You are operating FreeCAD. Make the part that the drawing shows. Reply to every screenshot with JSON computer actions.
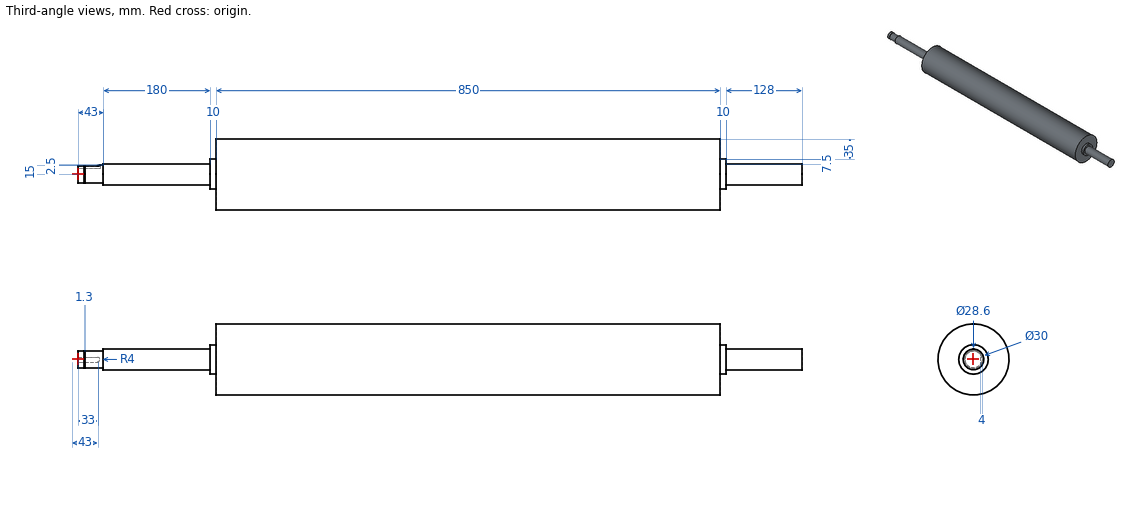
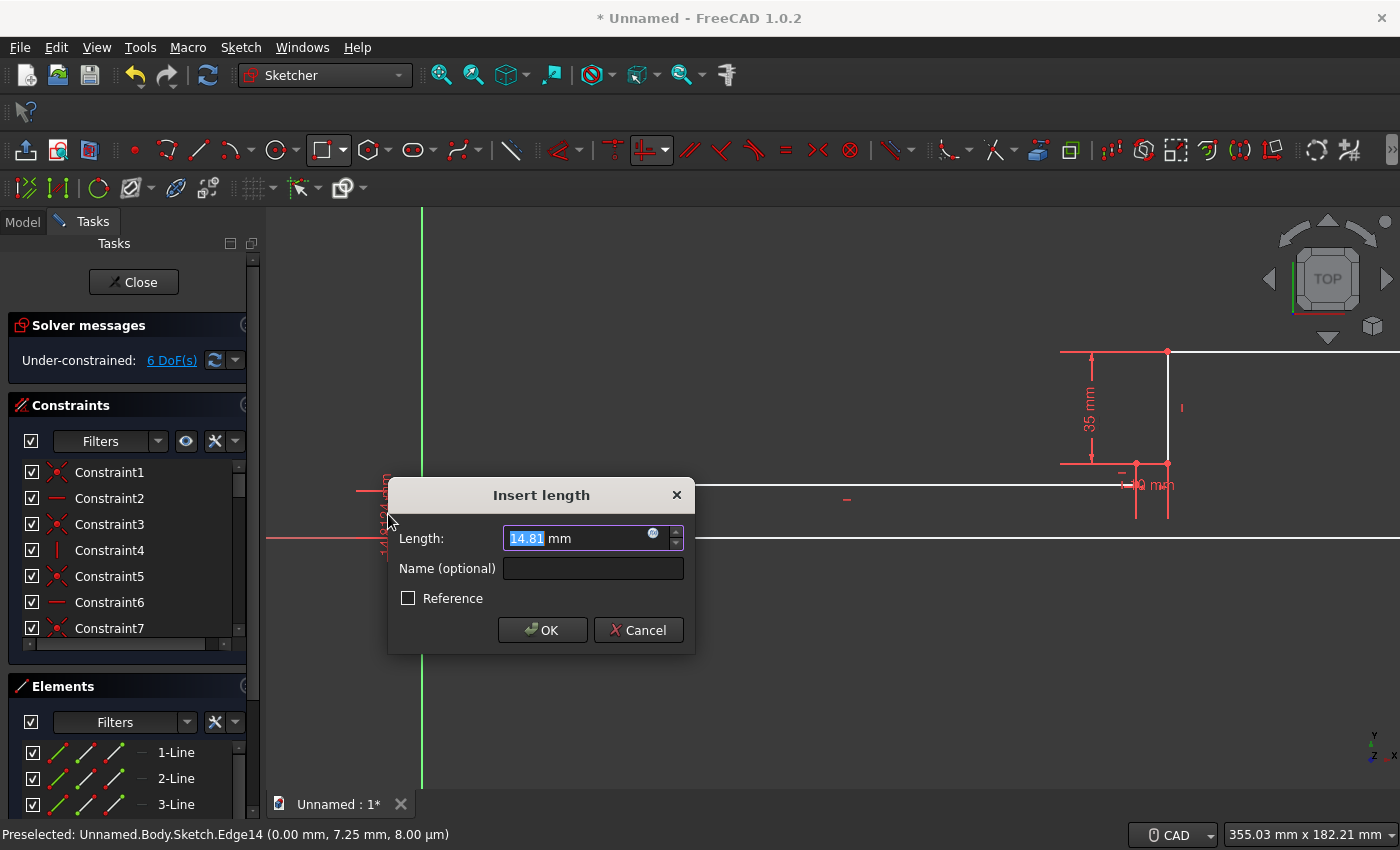
{"action": "type", "text": "15"}
{"action": "key", "text": "Return"}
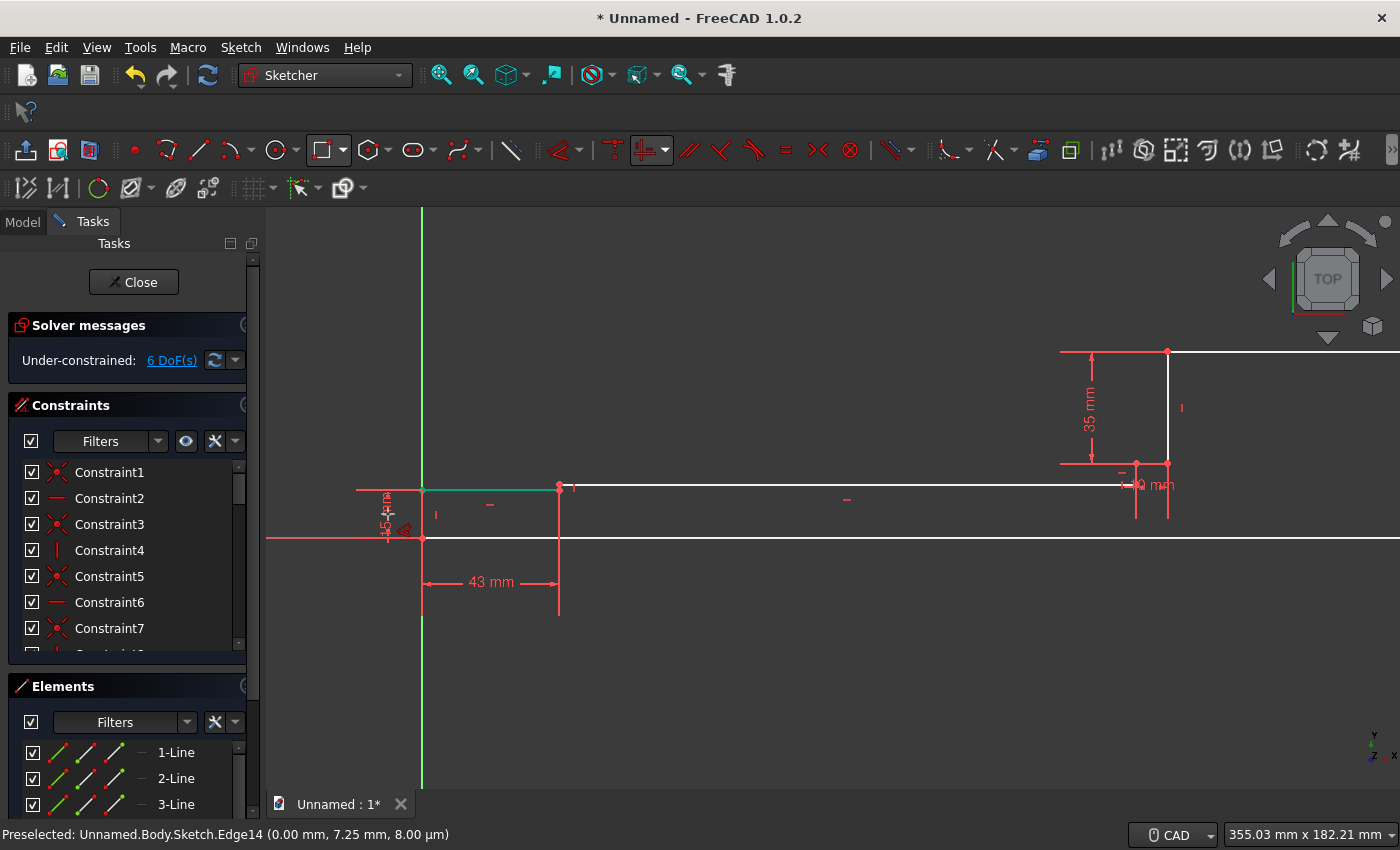
{"action": "scroll", "coordinate": [446, 509], "scroll_direction": "down", "scroll_amount": 9}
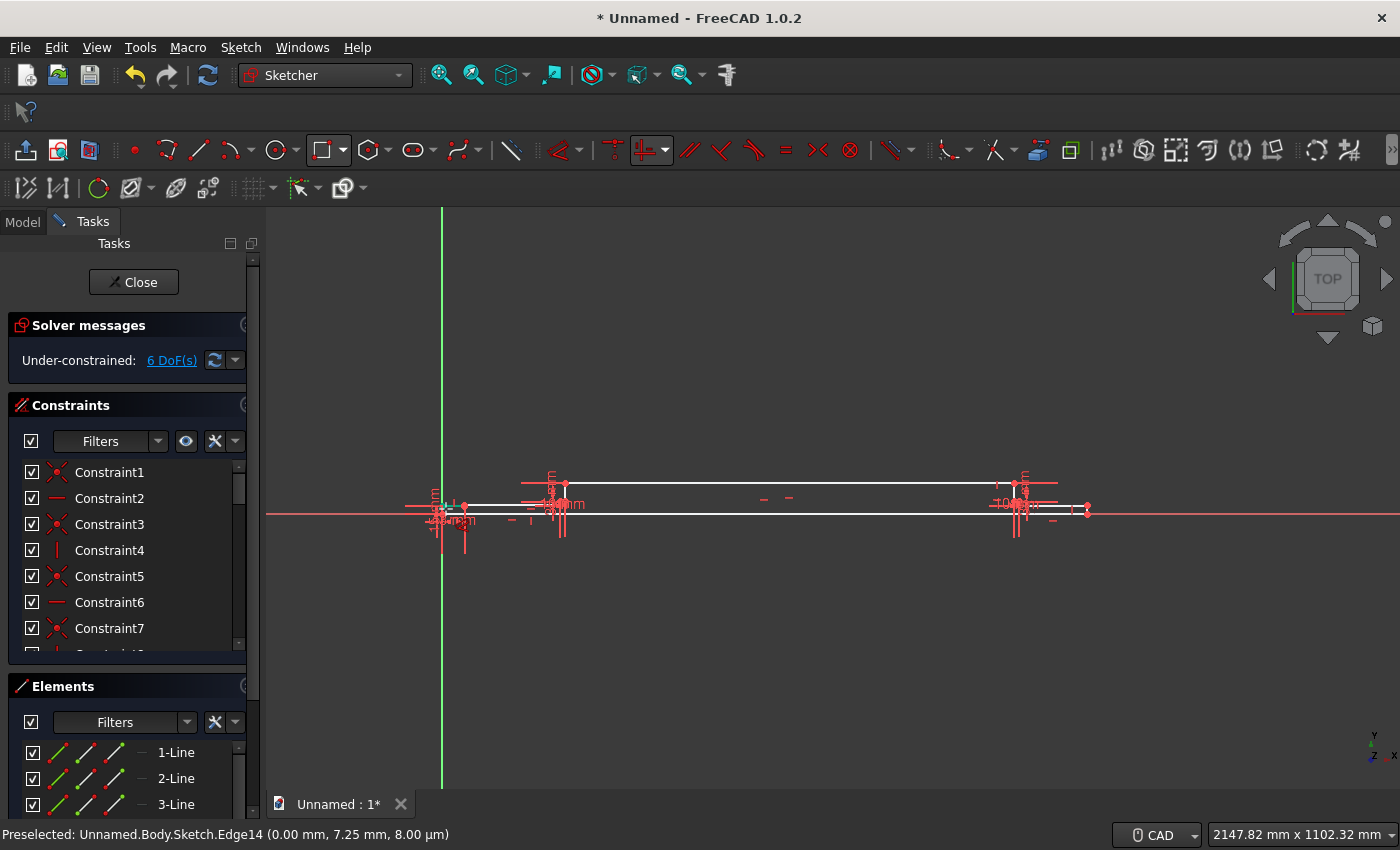
{"action": "scroll", "coordinate": [1067, 506], "scroll_direction": "up", "scroll_amount": 3}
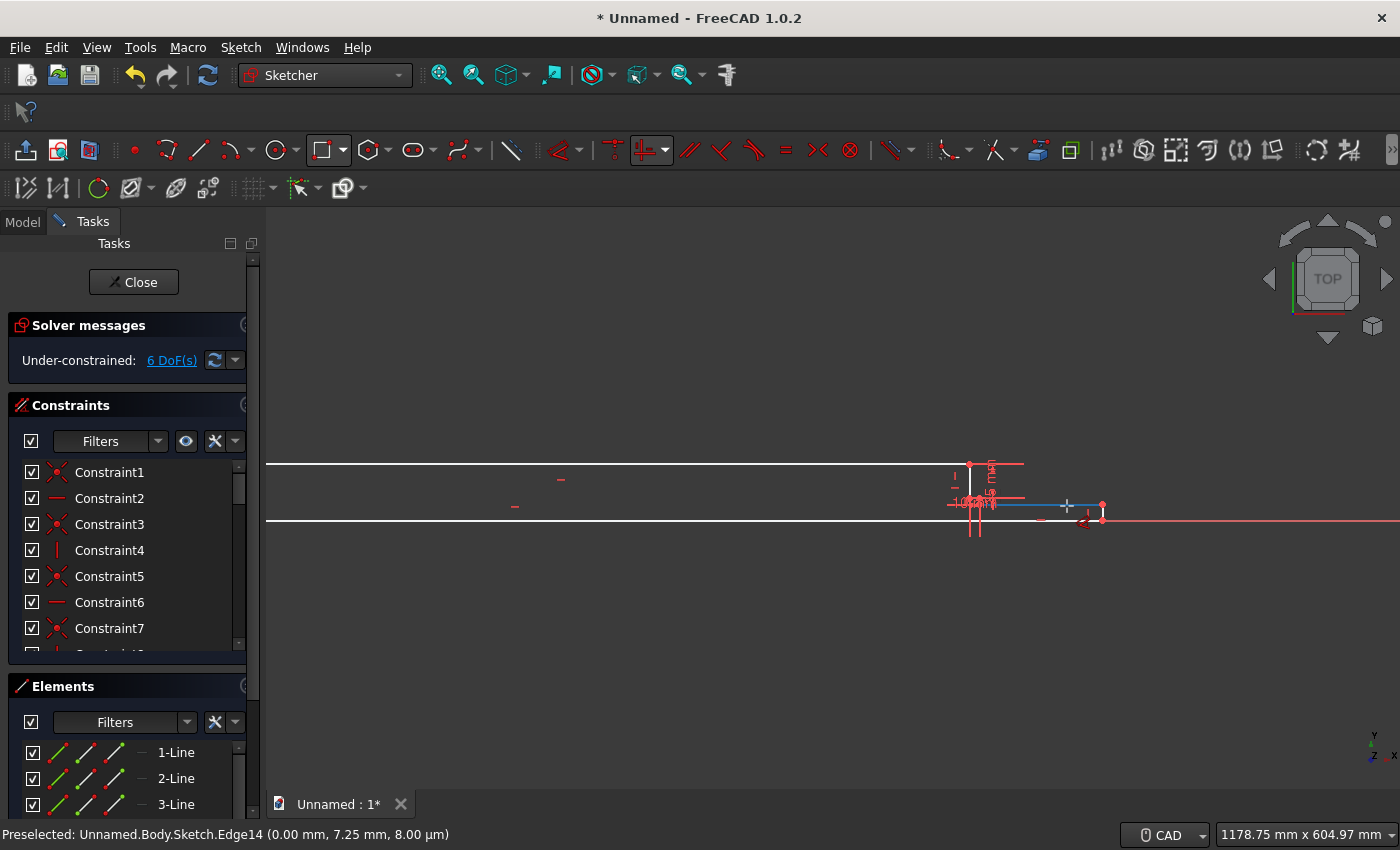
{"action": "left_click", "coordinate": [1066, 505]}
{"action": "left_click", "coordinate": [1041, 539]}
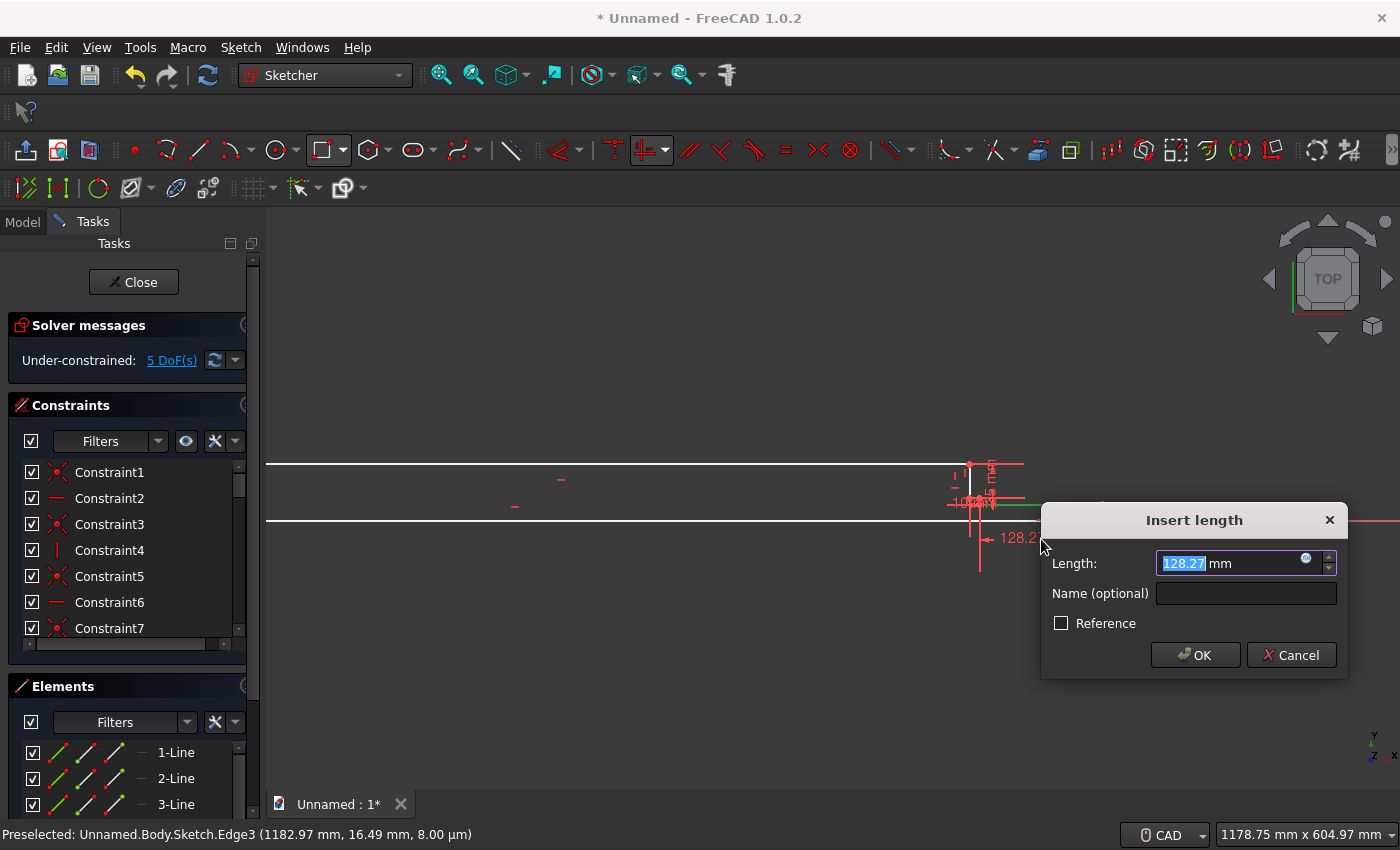
{"action": "type", "text": "128"}
{"action": "key", "text": "Return"}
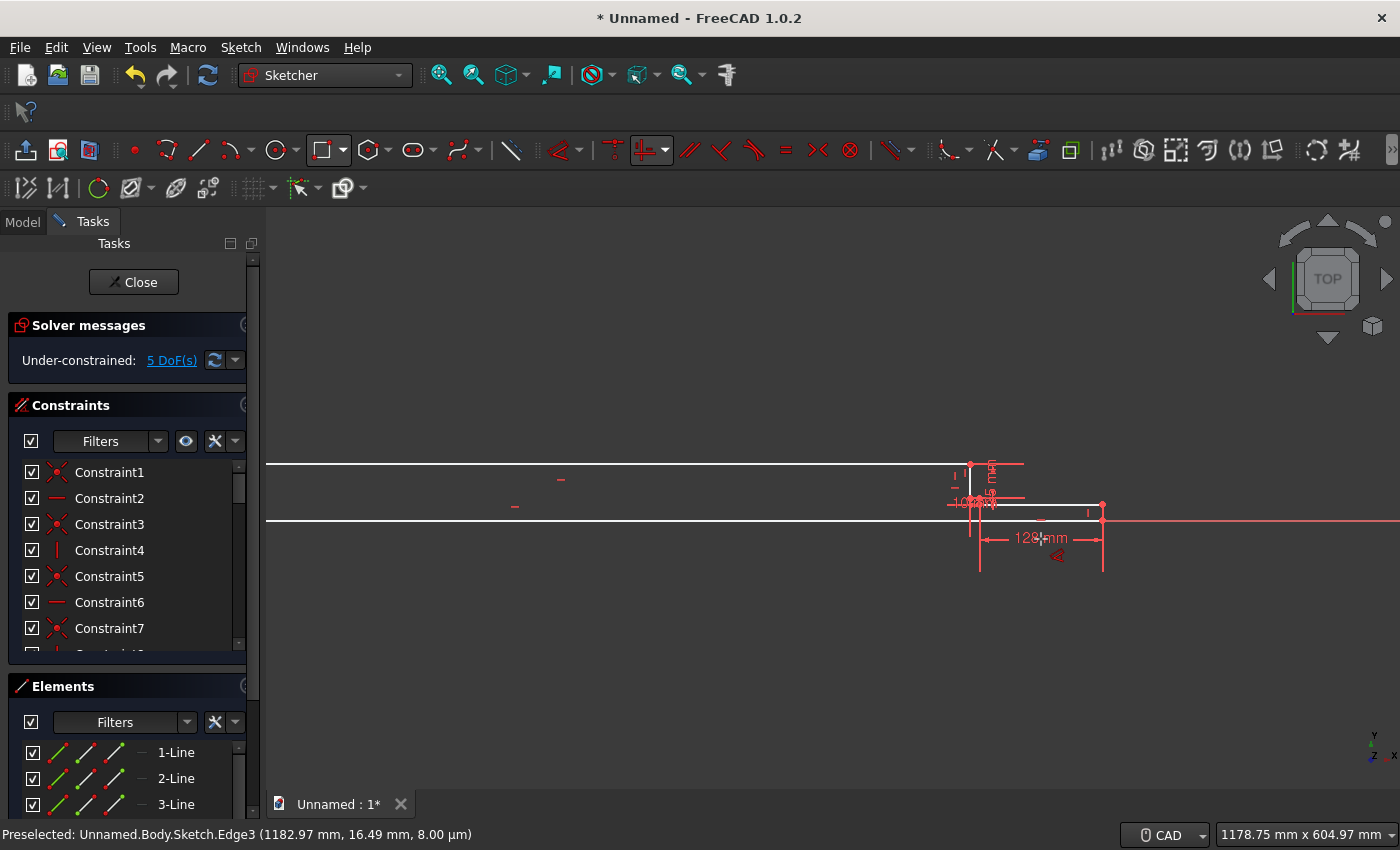
{"action": "scroll", "coordinate": [980, 501], "scroll_direction": "up", "scroll_amount": 9}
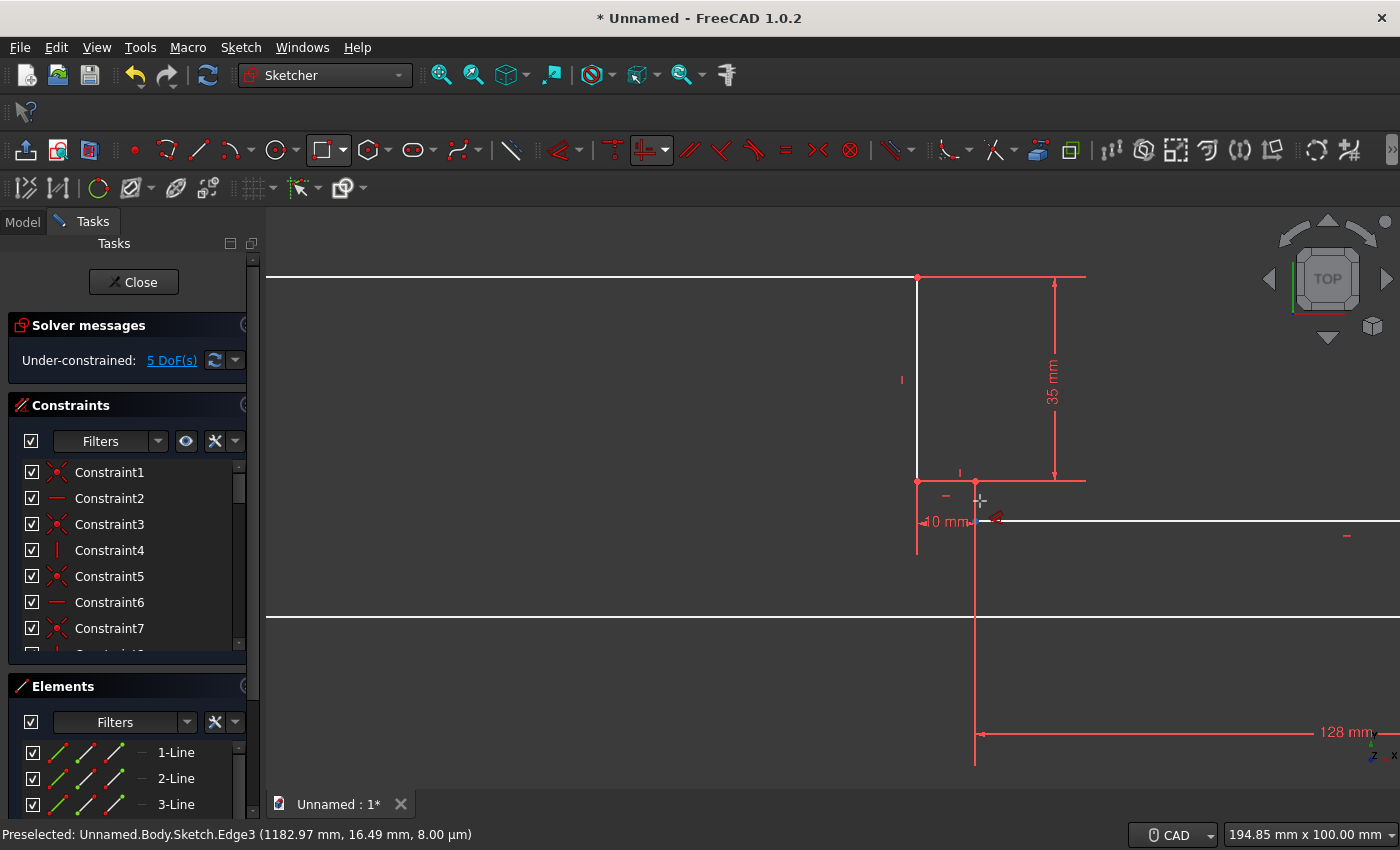
{"action": "left_click", "coordinate": [975, 501]}
{"action": "left_click", "coordinate": [1009, 492]}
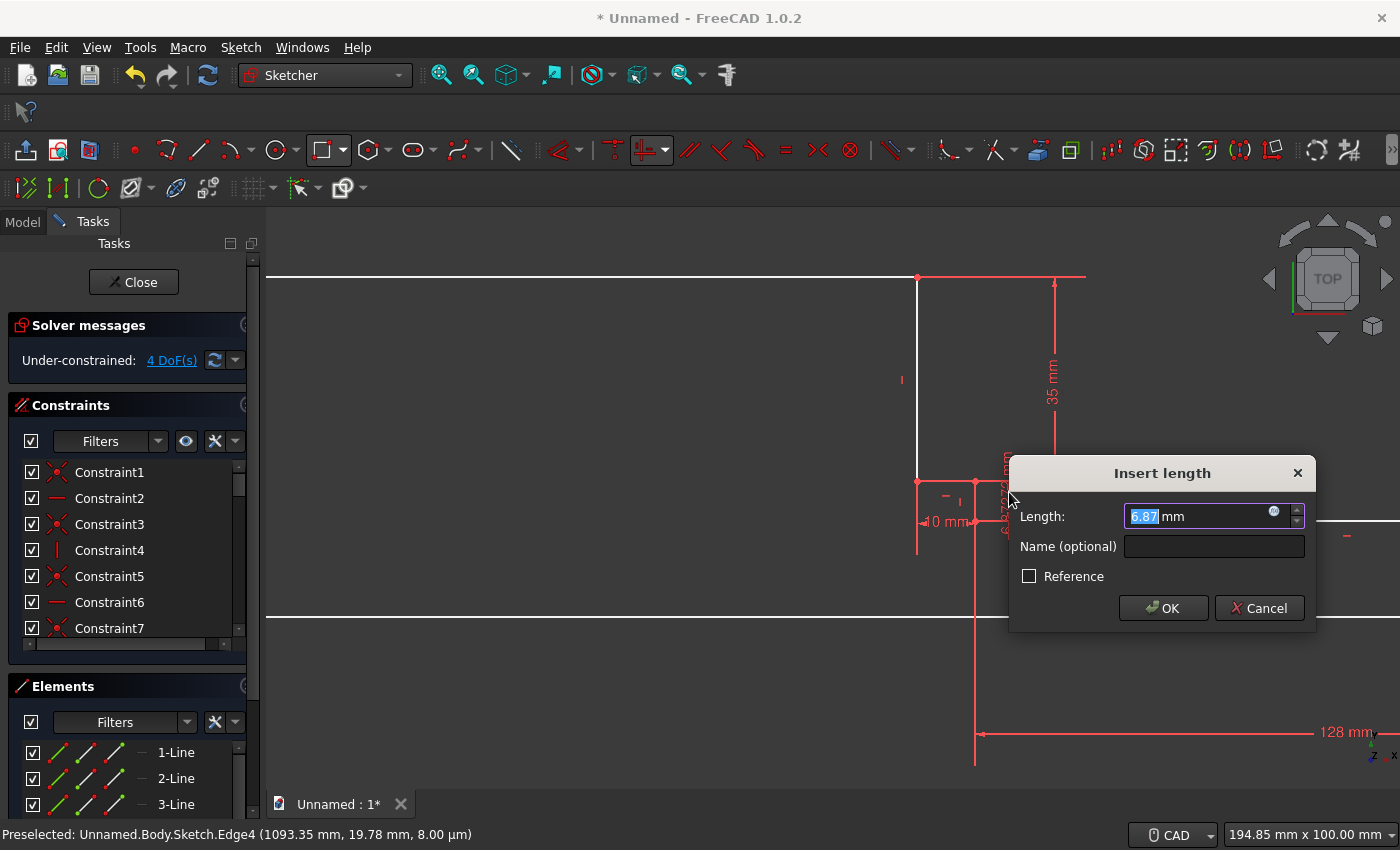
{"action": "type", "text": "7.5"}
{"action": "key", "text": "Return"}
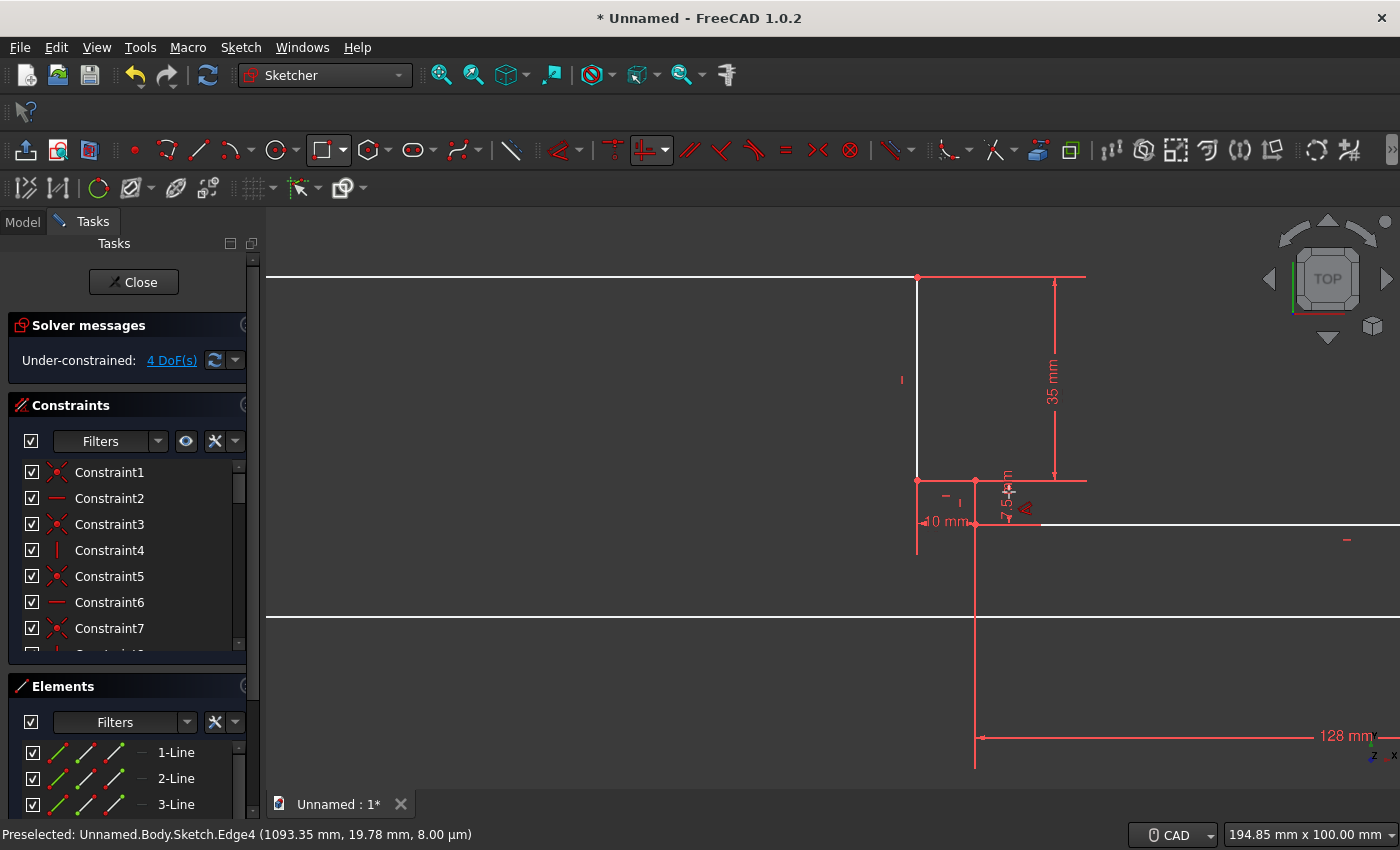
{"action": "scroll", "coordinate": [1024, 504], "scroll_direction": "down", "scroll_amount": 12}